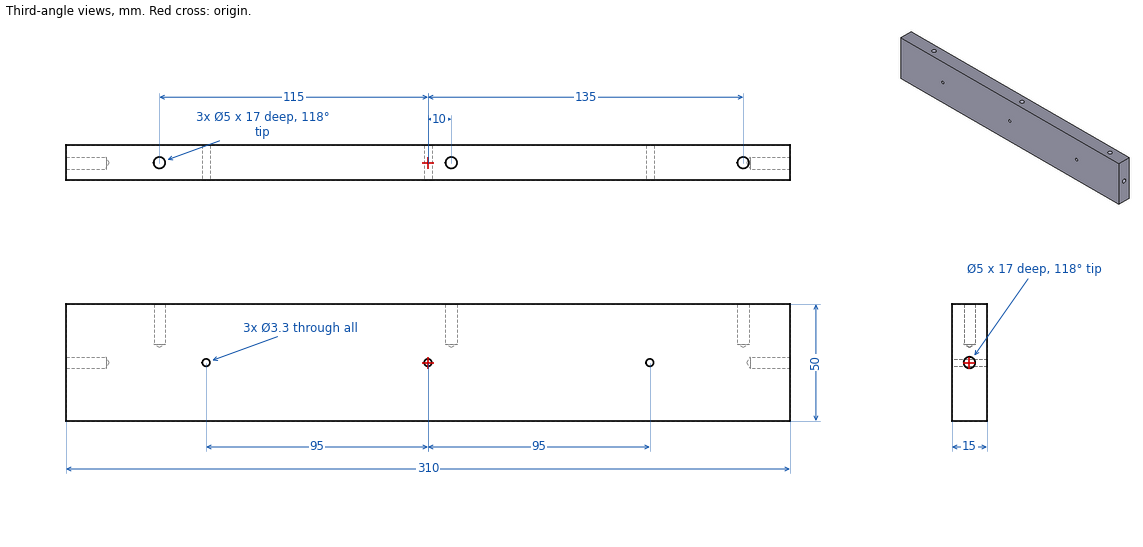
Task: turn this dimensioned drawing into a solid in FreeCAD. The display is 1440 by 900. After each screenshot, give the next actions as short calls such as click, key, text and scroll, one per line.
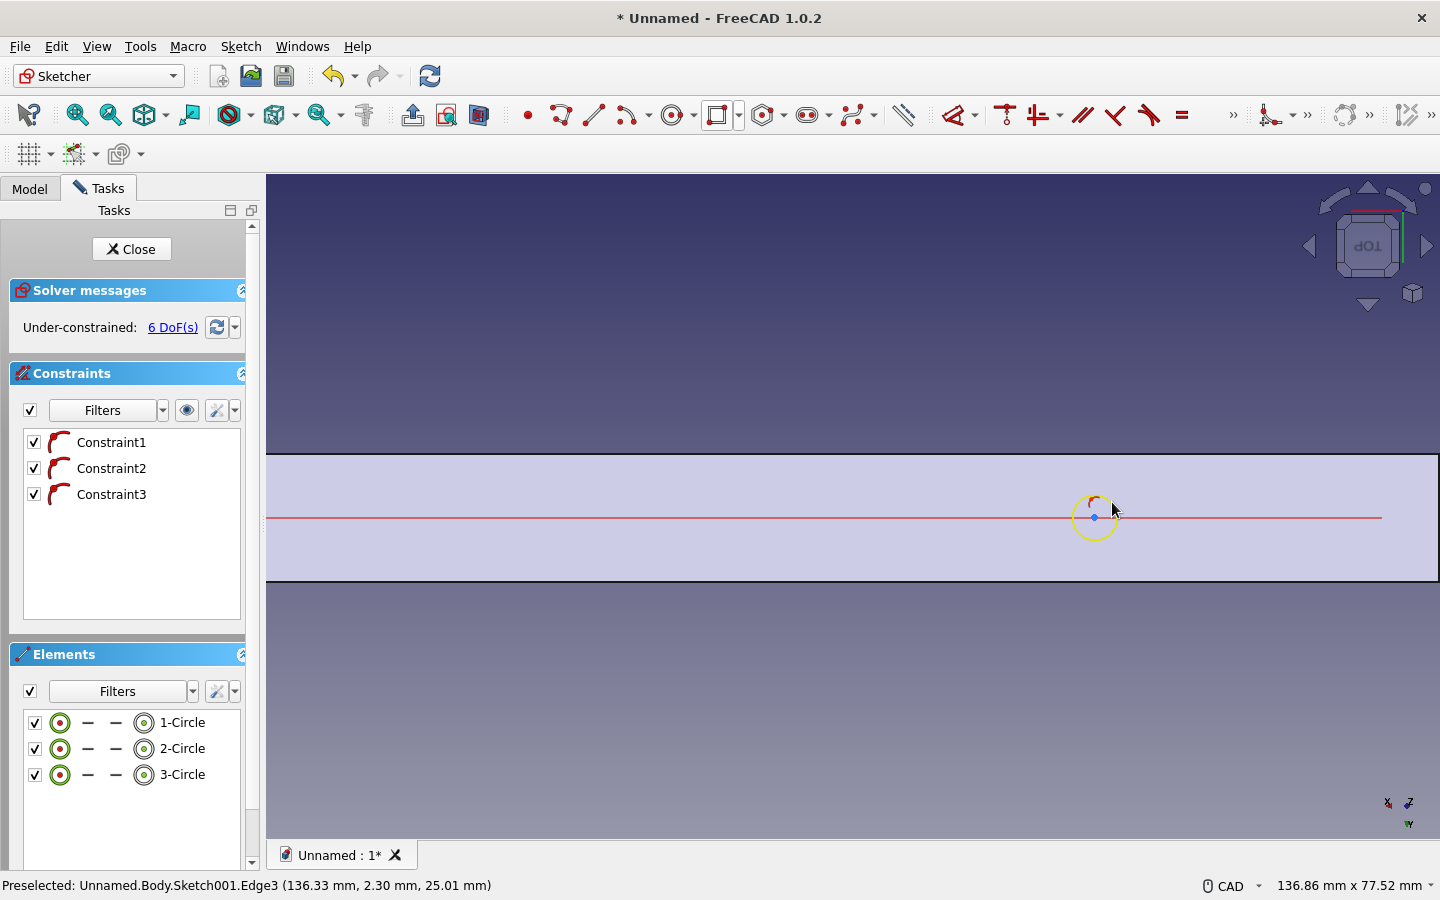
click(1111, 502)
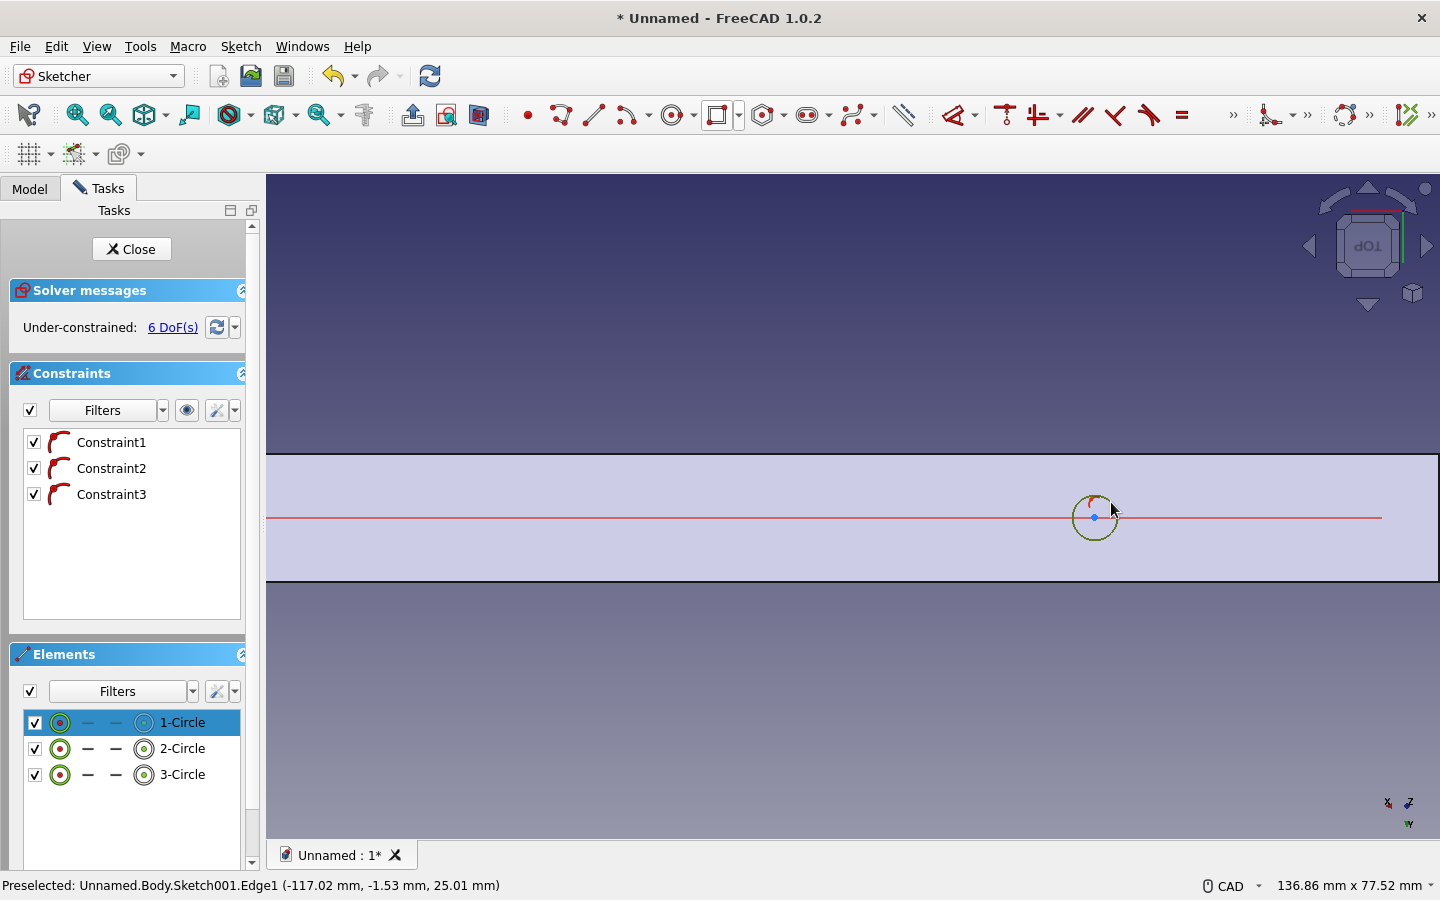
scroll(1113, 502, down, 6)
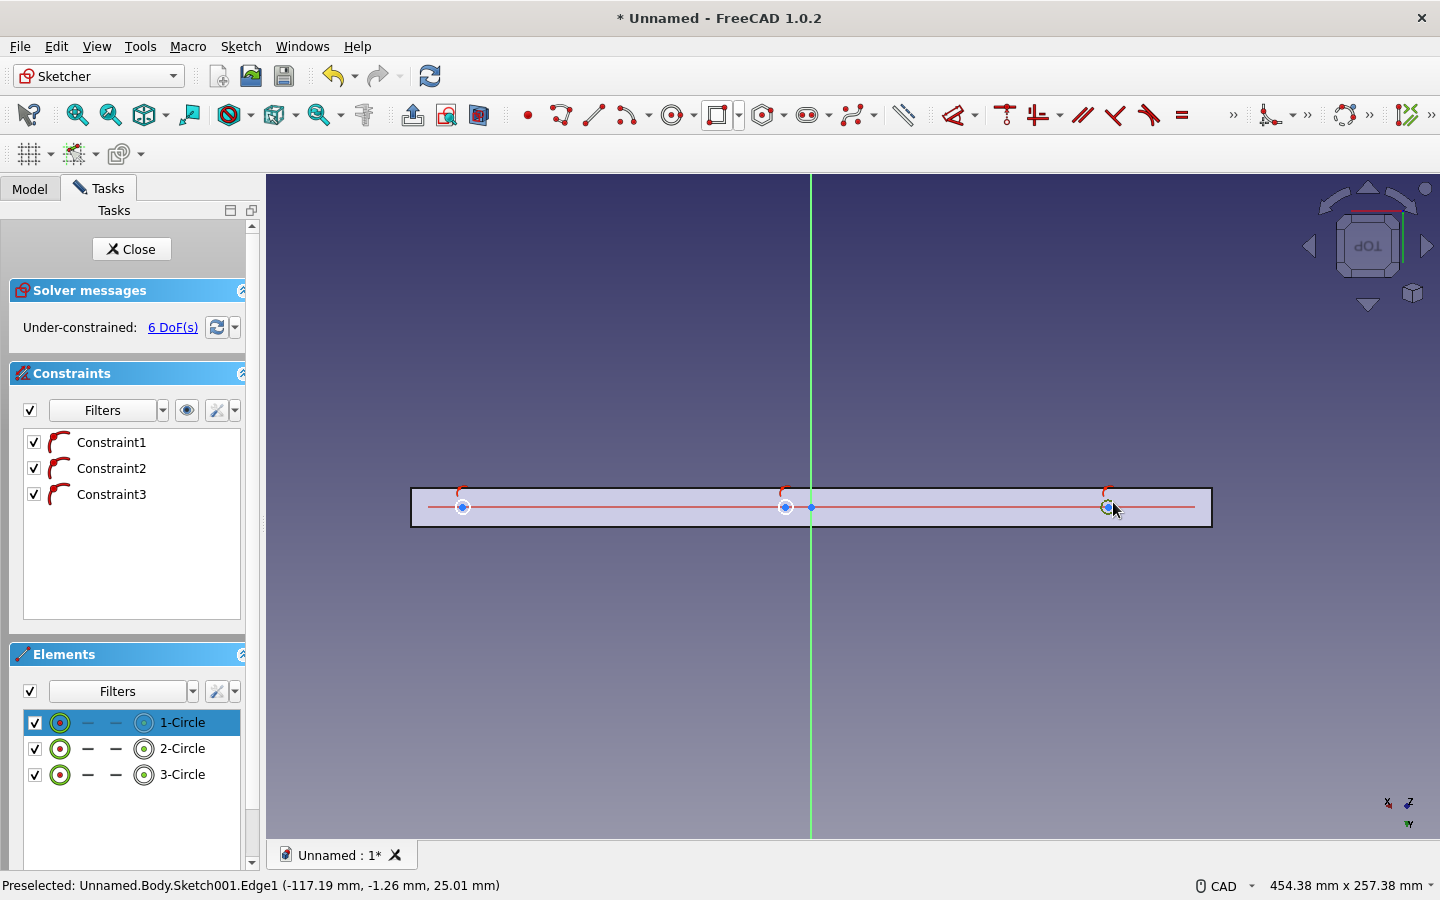
scroll(791, 502, up, 6)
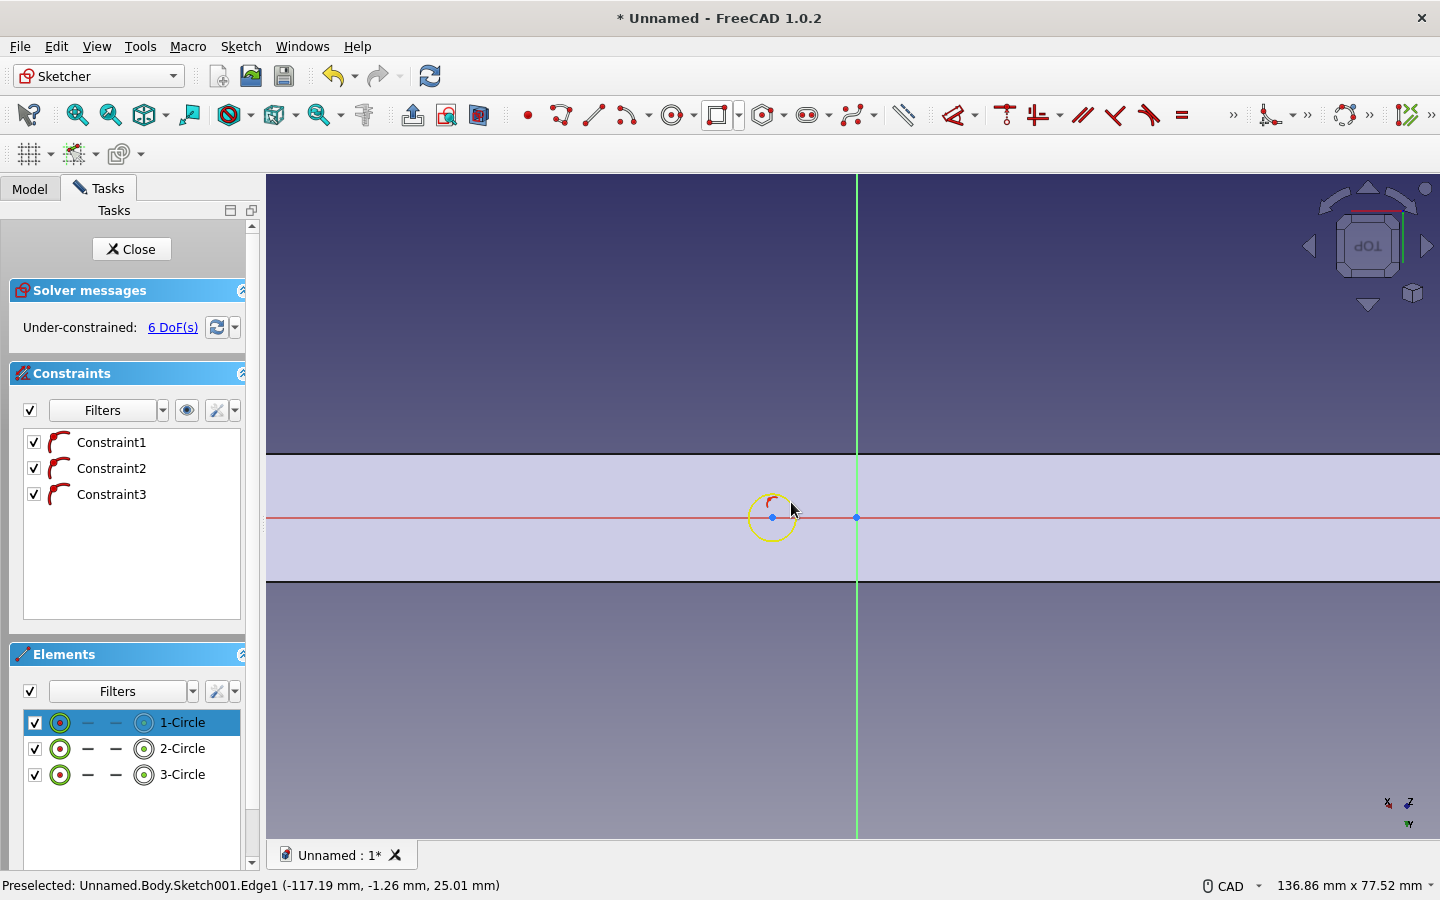
click(789, 501)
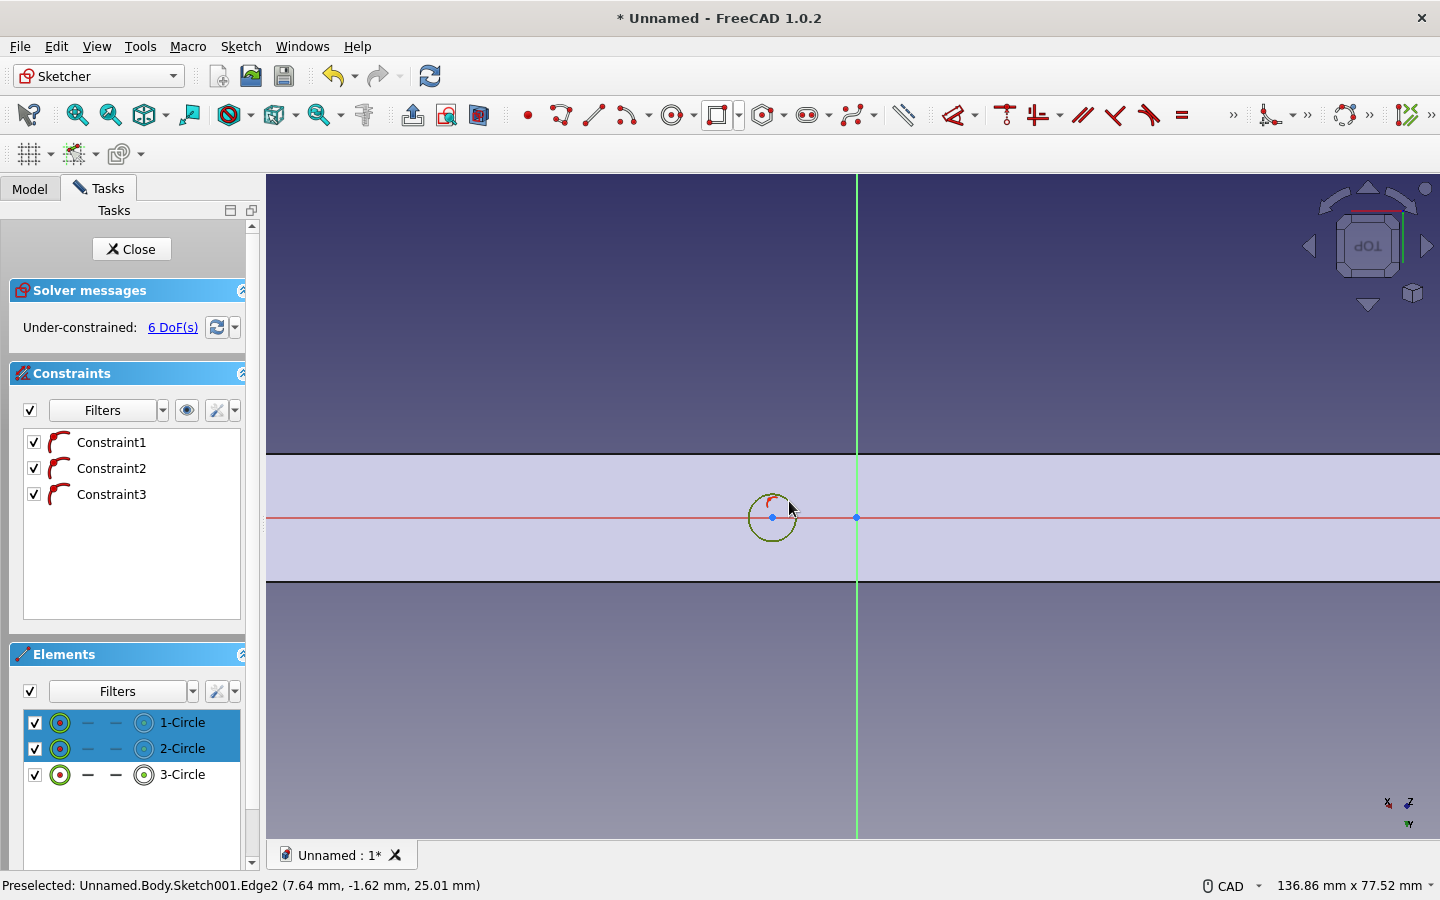
scroll(790, 502, down, 6)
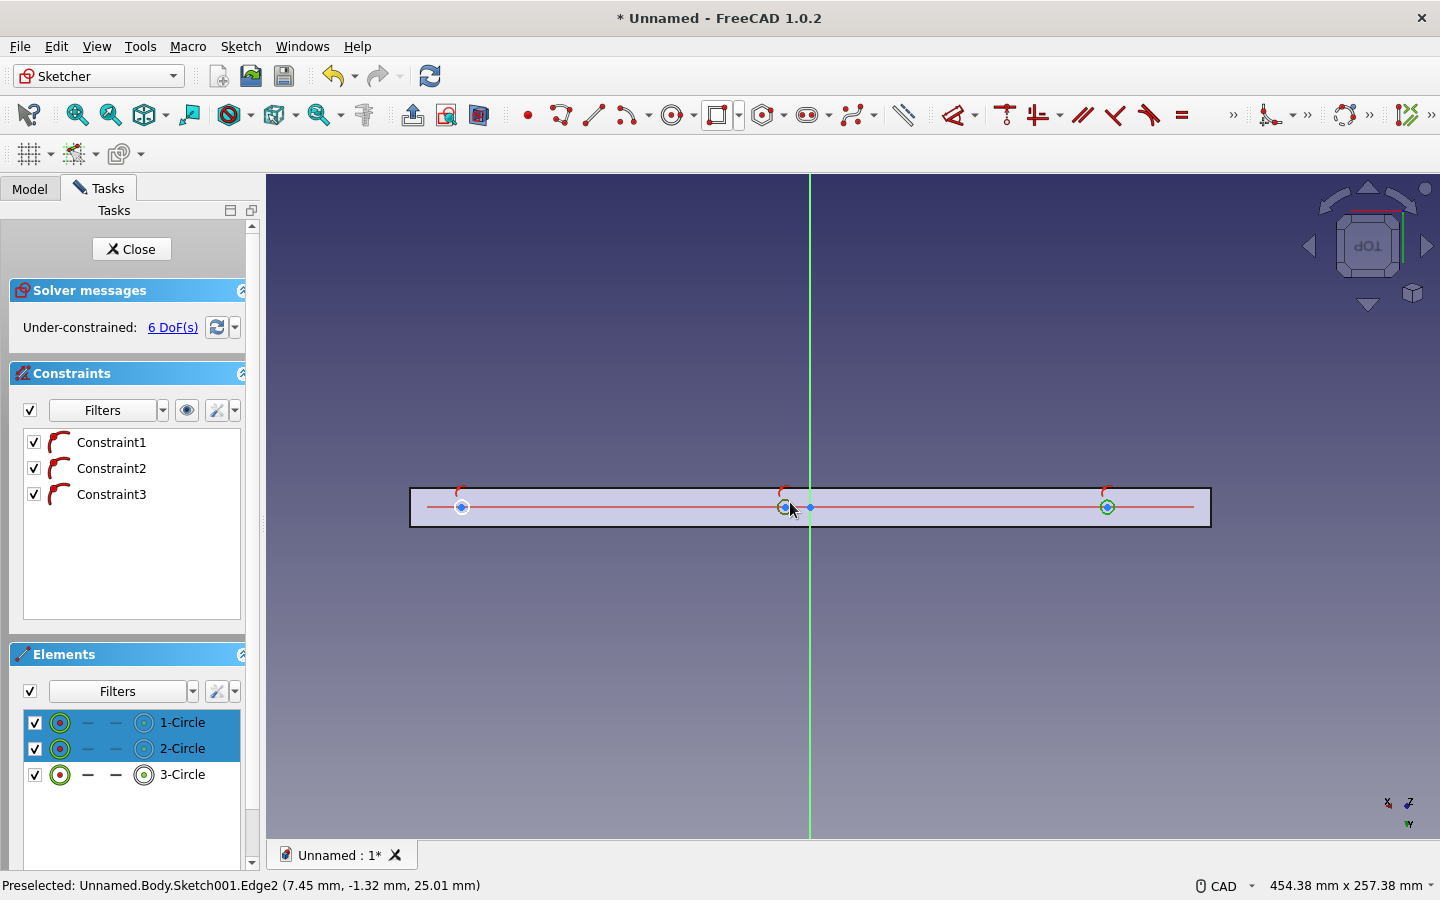
scroll(467, 502, up, 6)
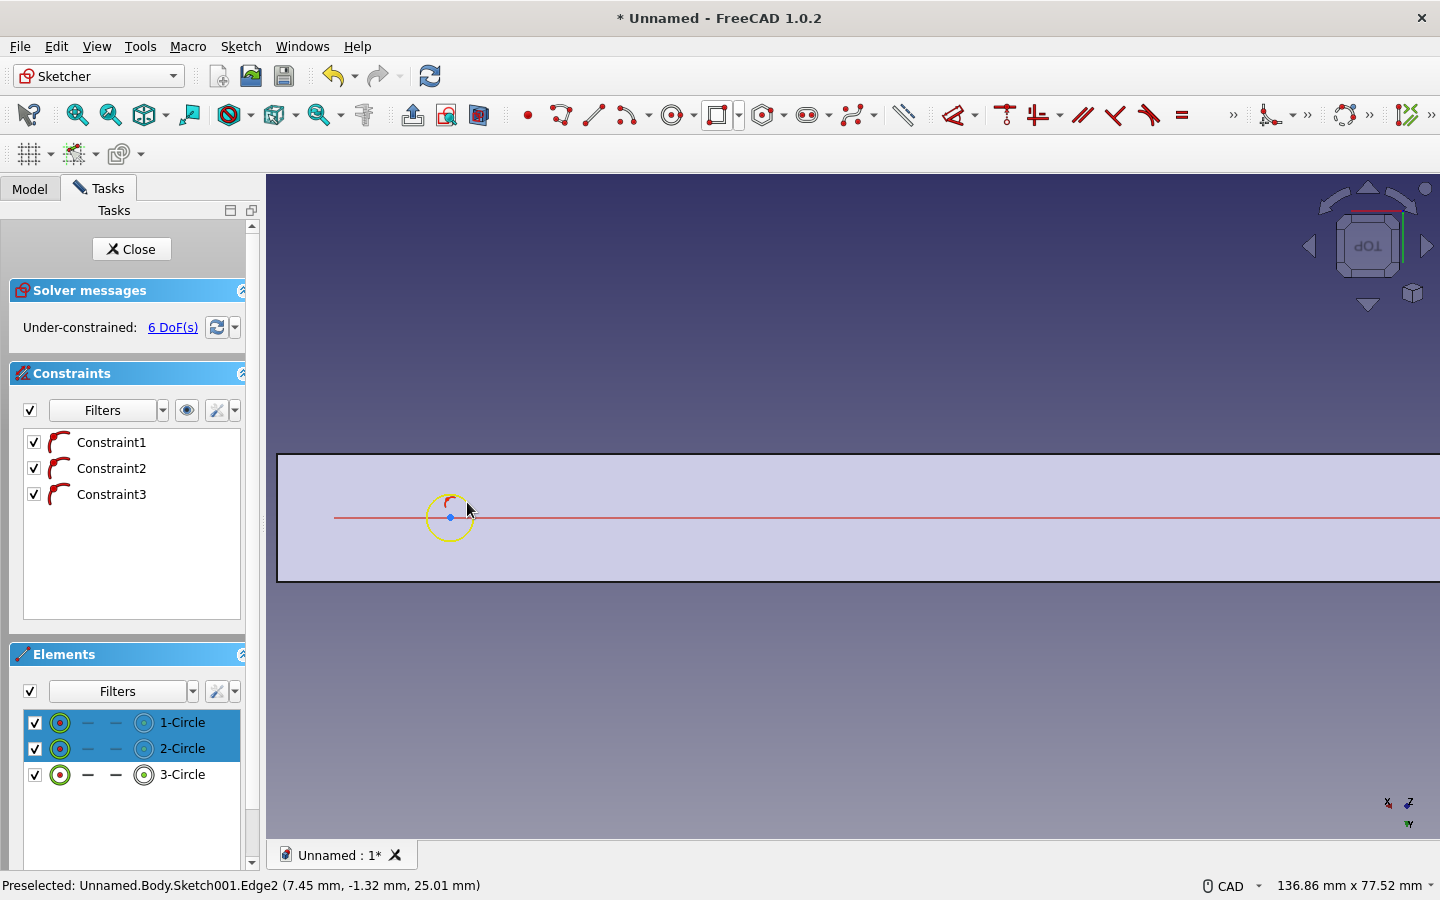
click(466, 501)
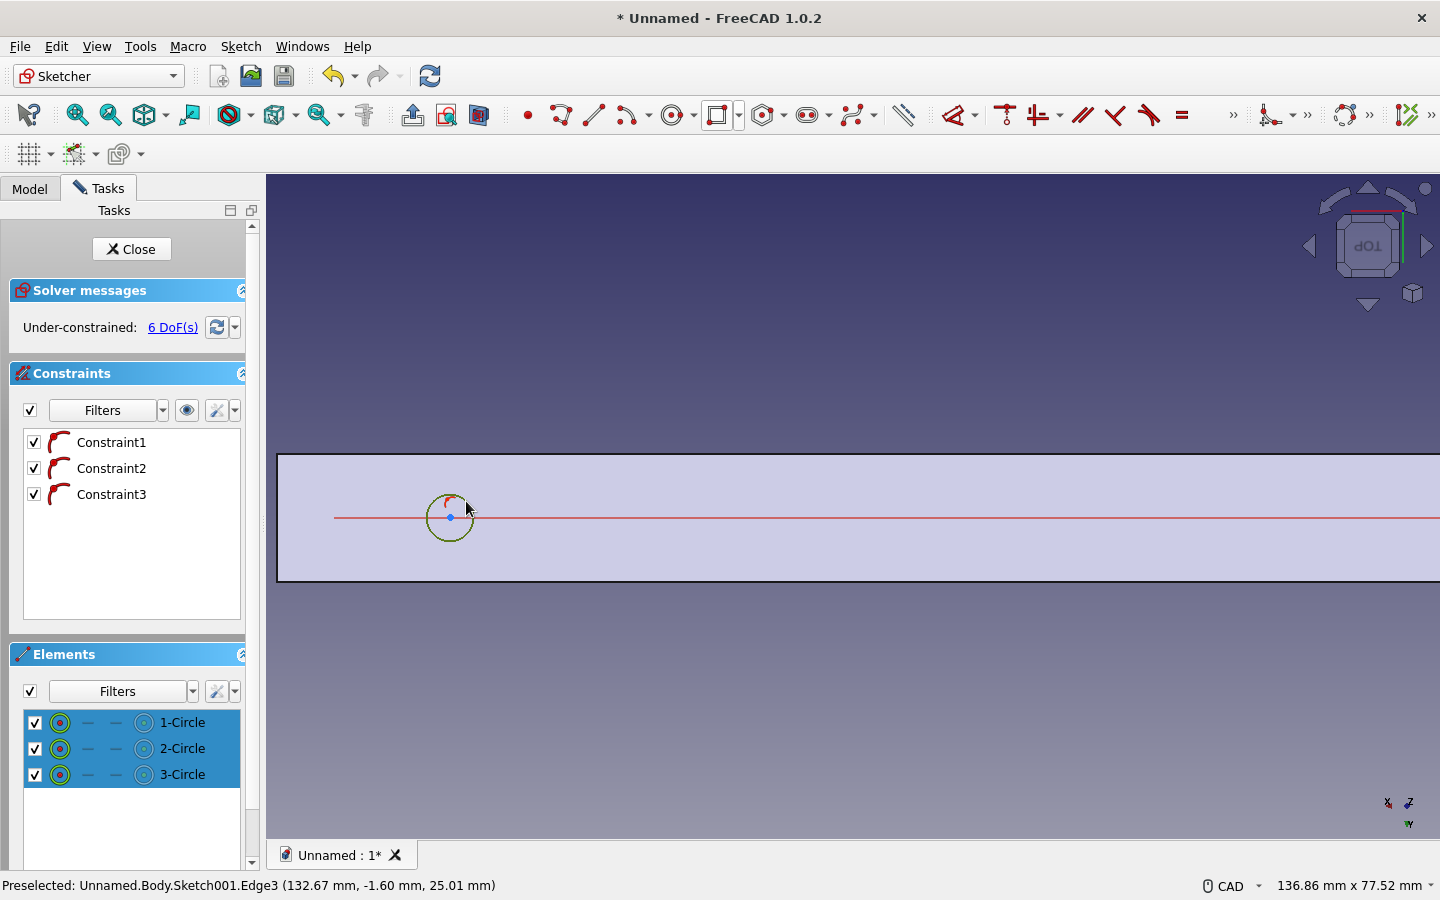
click(1182, 116)